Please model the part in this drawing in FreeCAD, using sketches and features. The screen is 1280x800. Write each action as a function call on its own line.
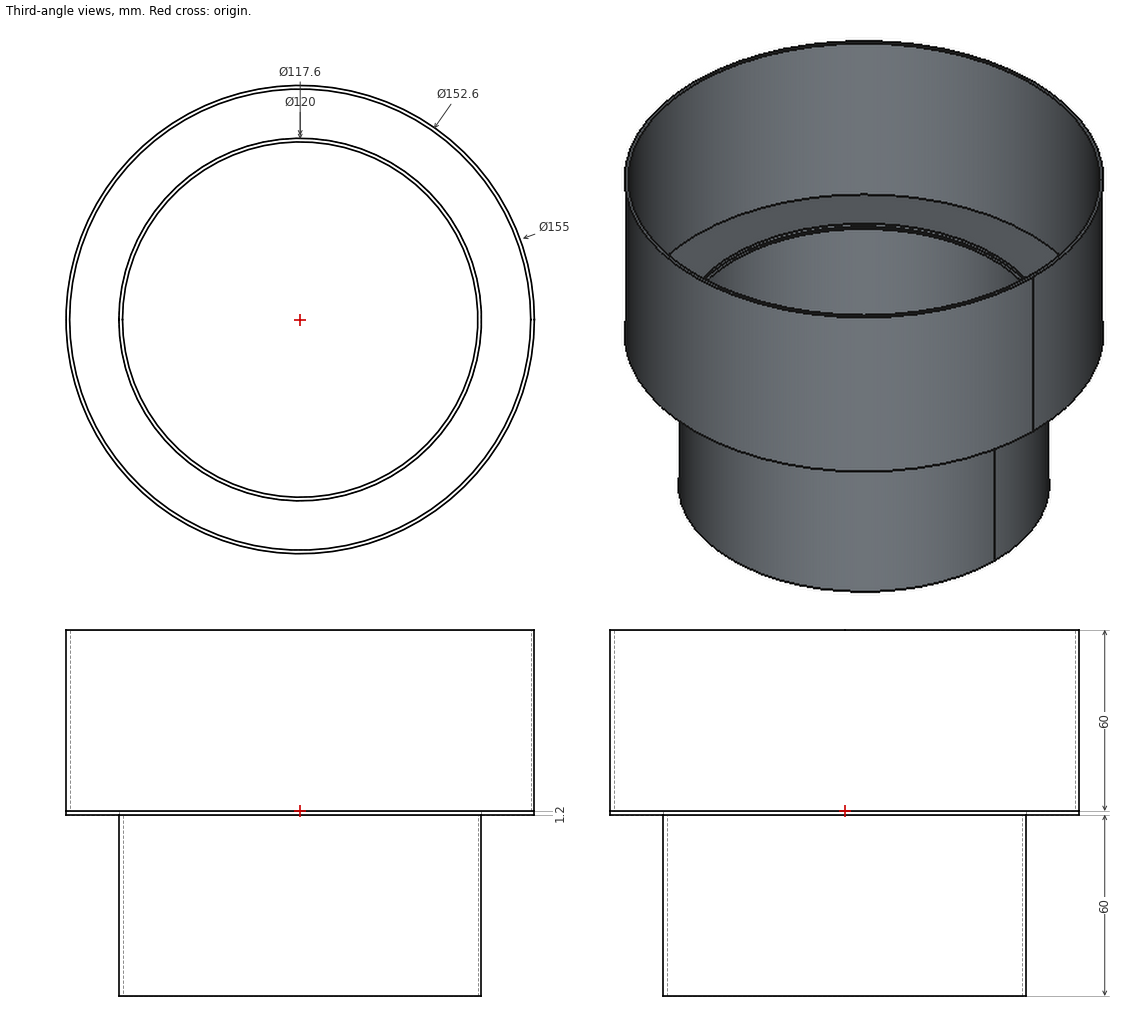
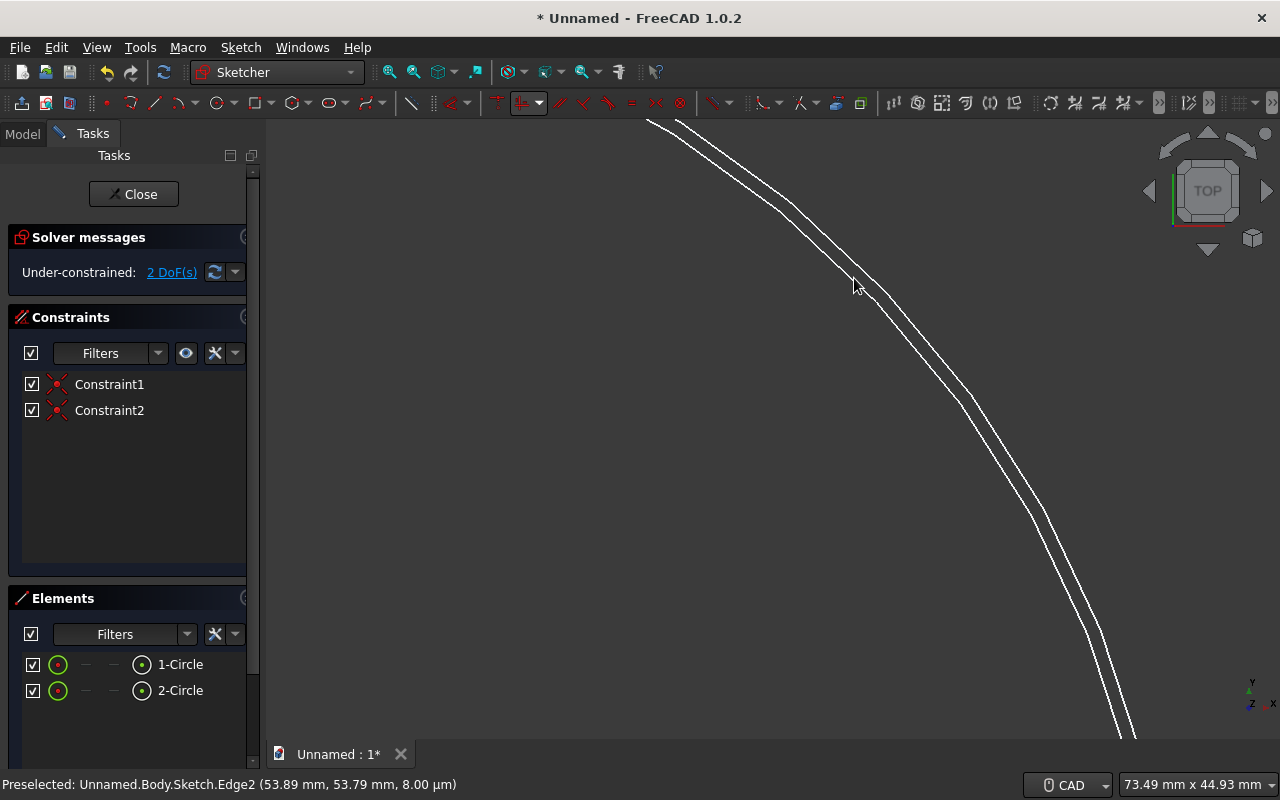
click(450, 104)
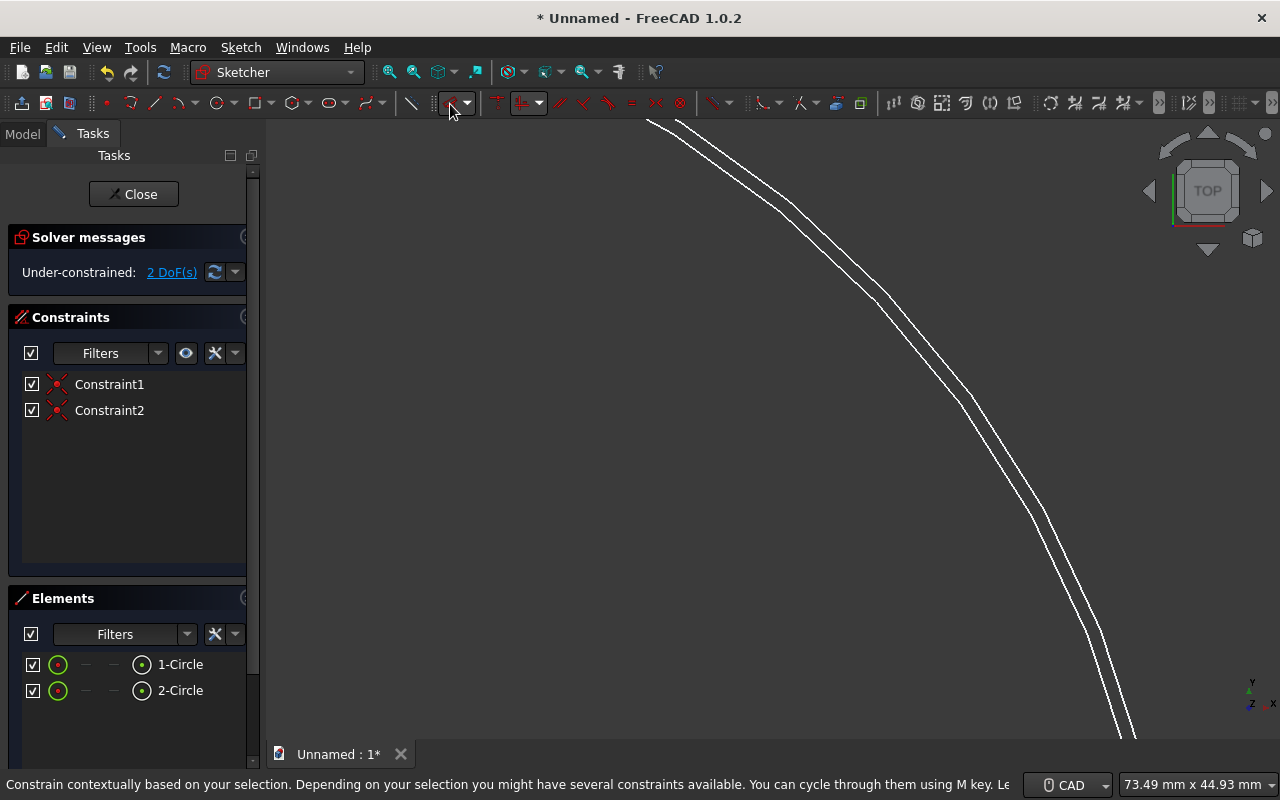
click(861, 266)
click(884, 243)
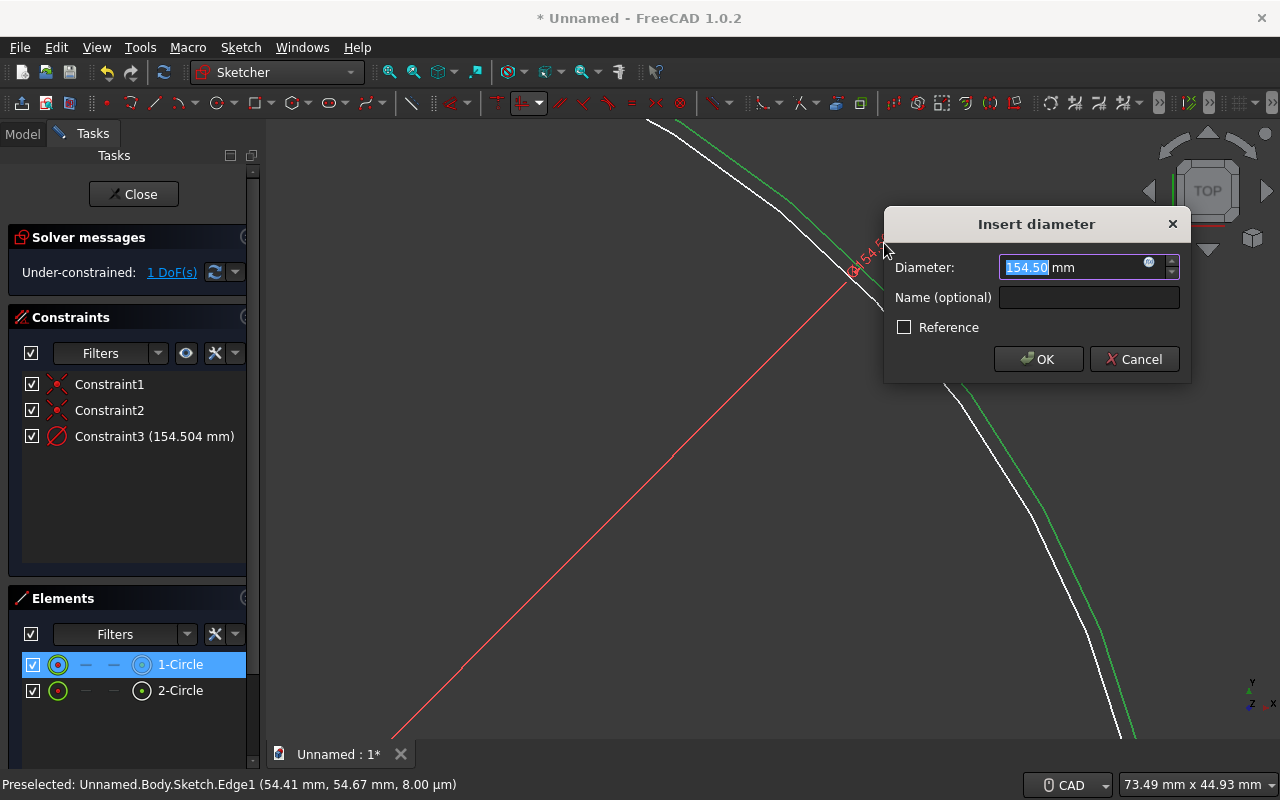
text(155)
key(Return)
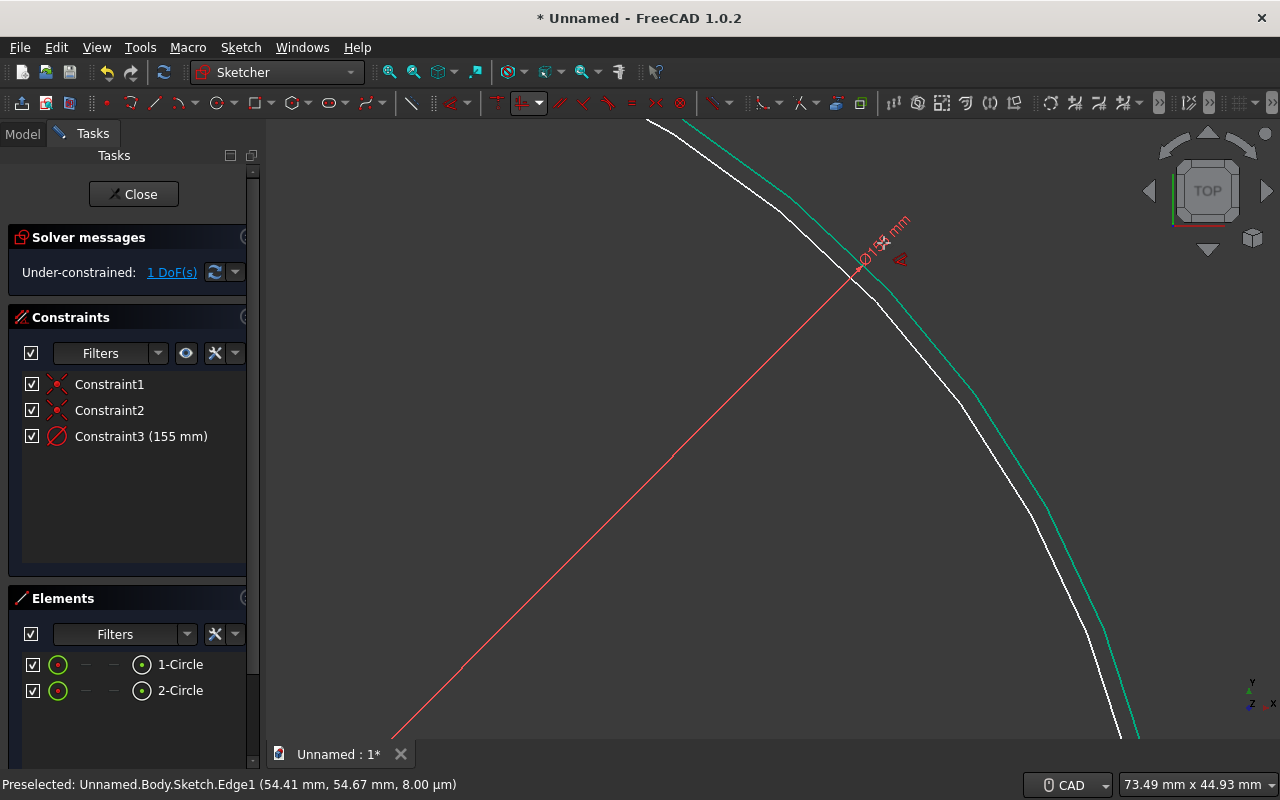
click(851, 276)
click(907, 219)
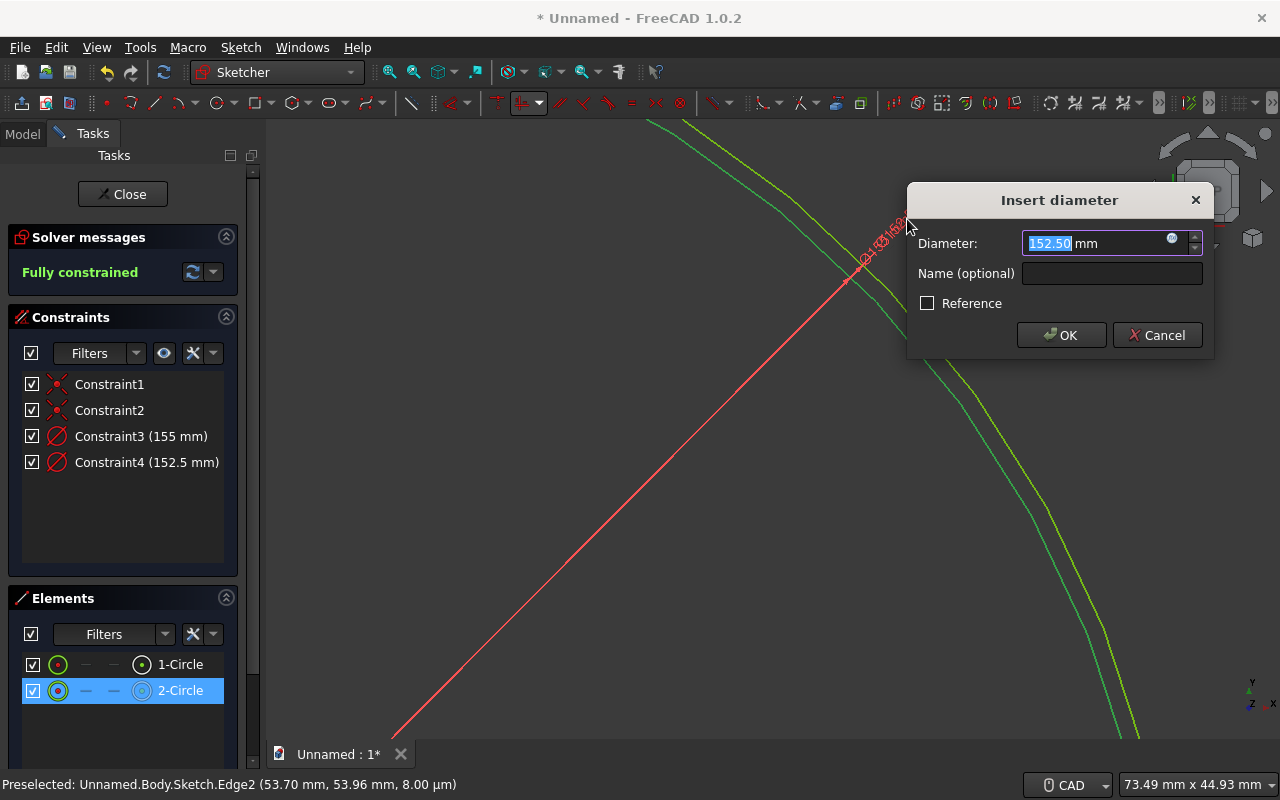
text(152.6)
key(Return)
key(Escape)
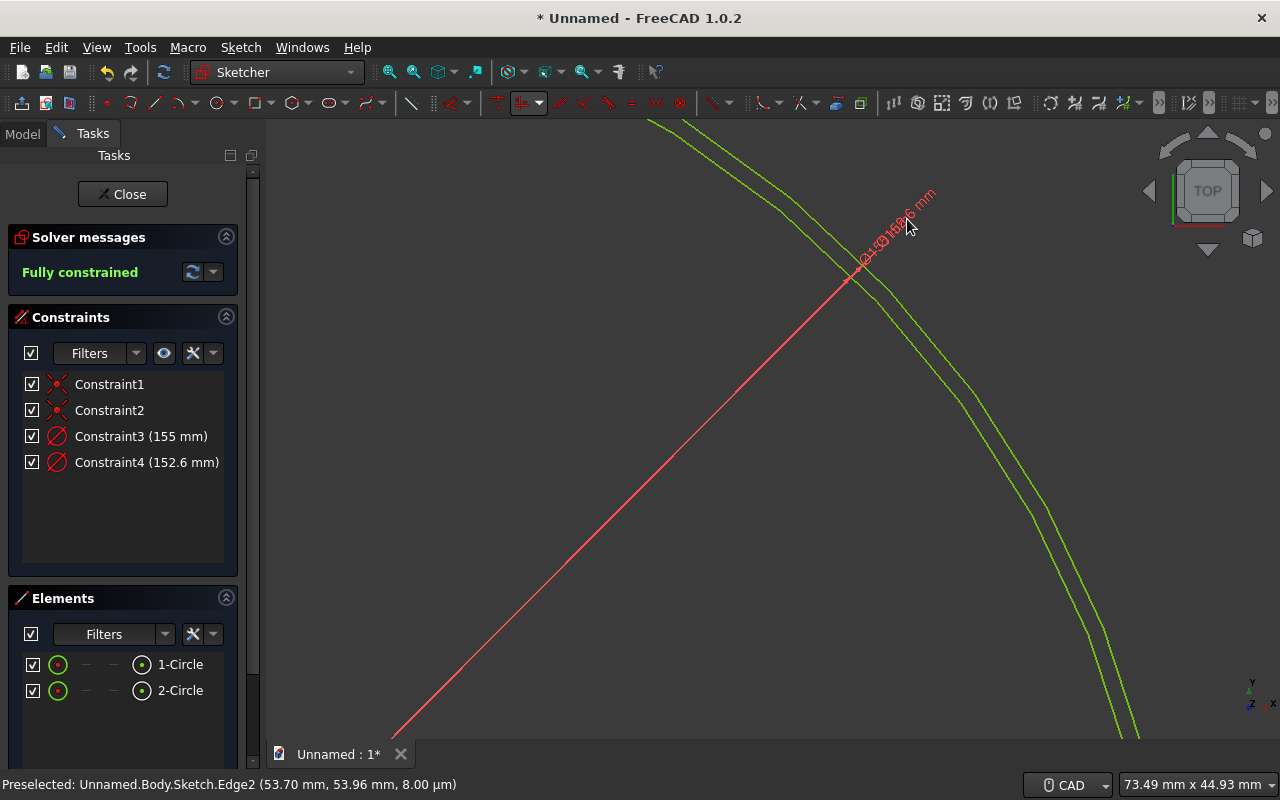
click(123, 194)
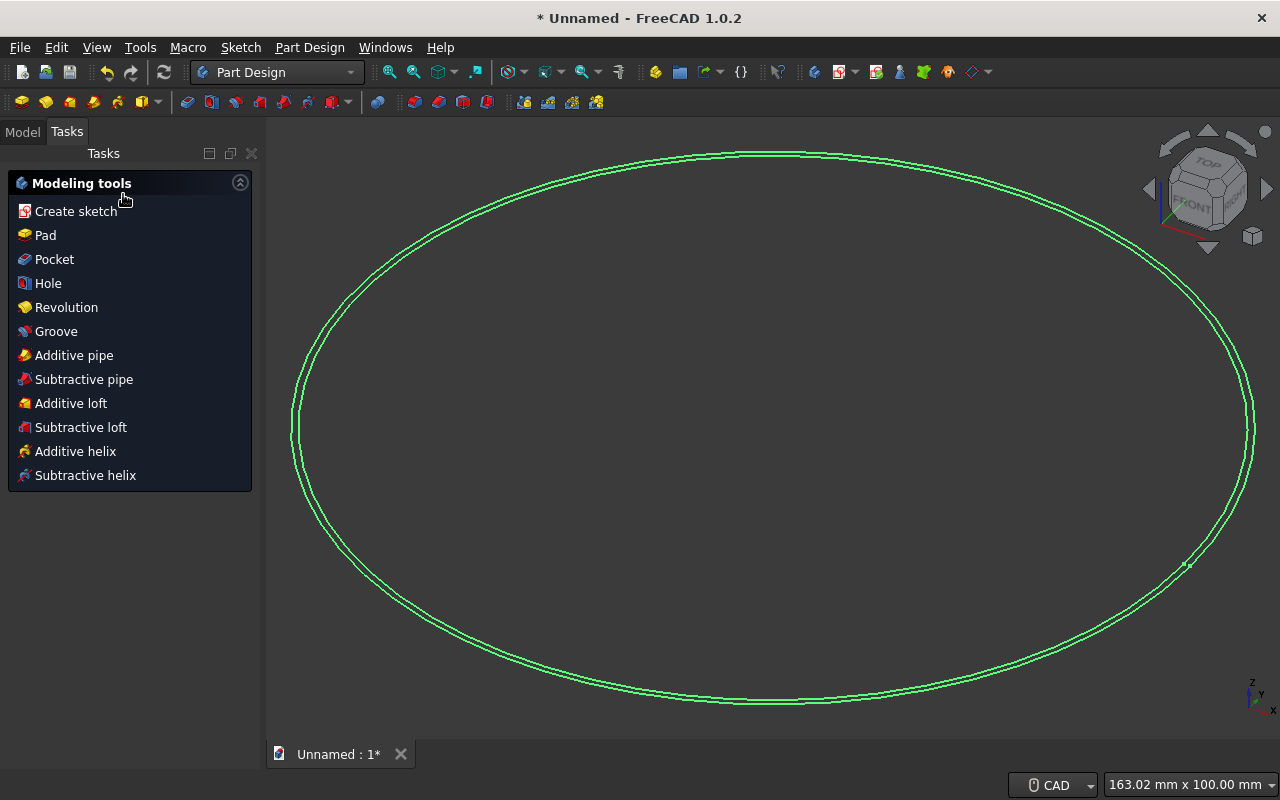
click(22, 102)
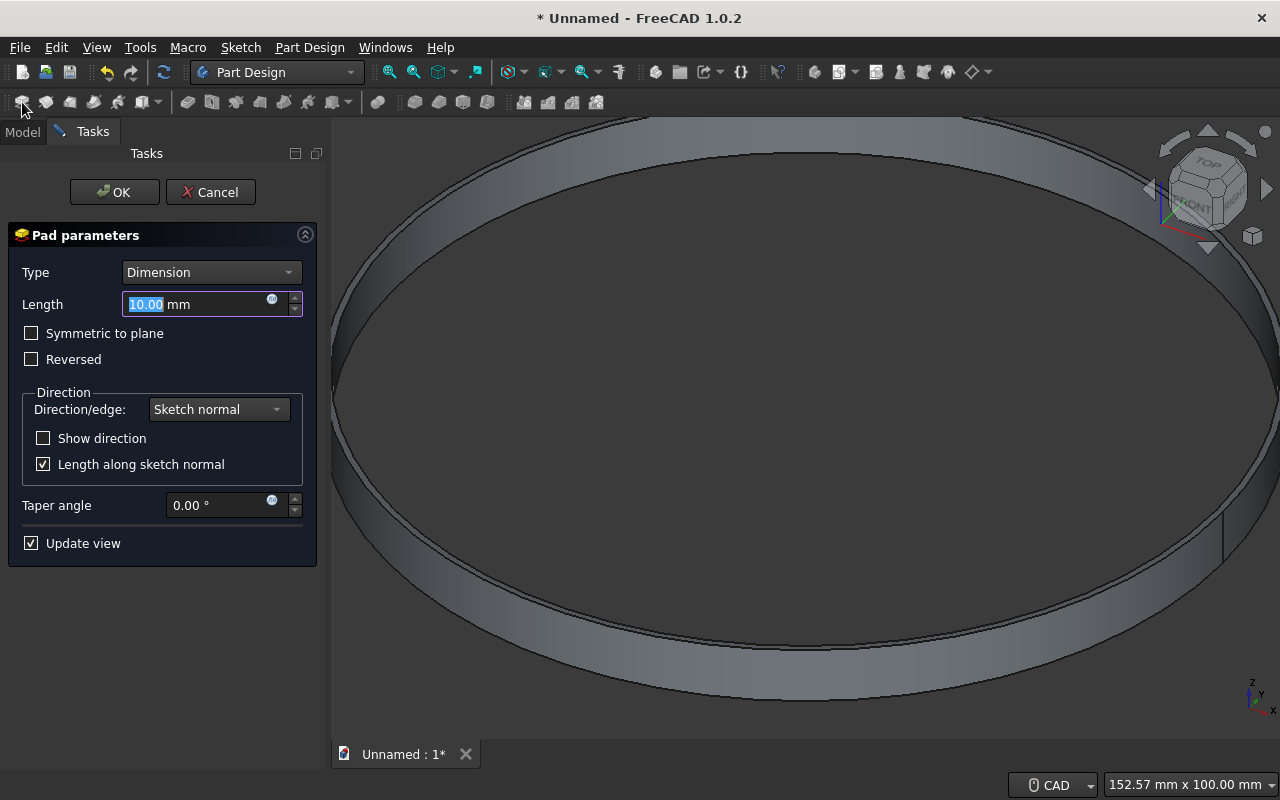
text(60)
key(Tab)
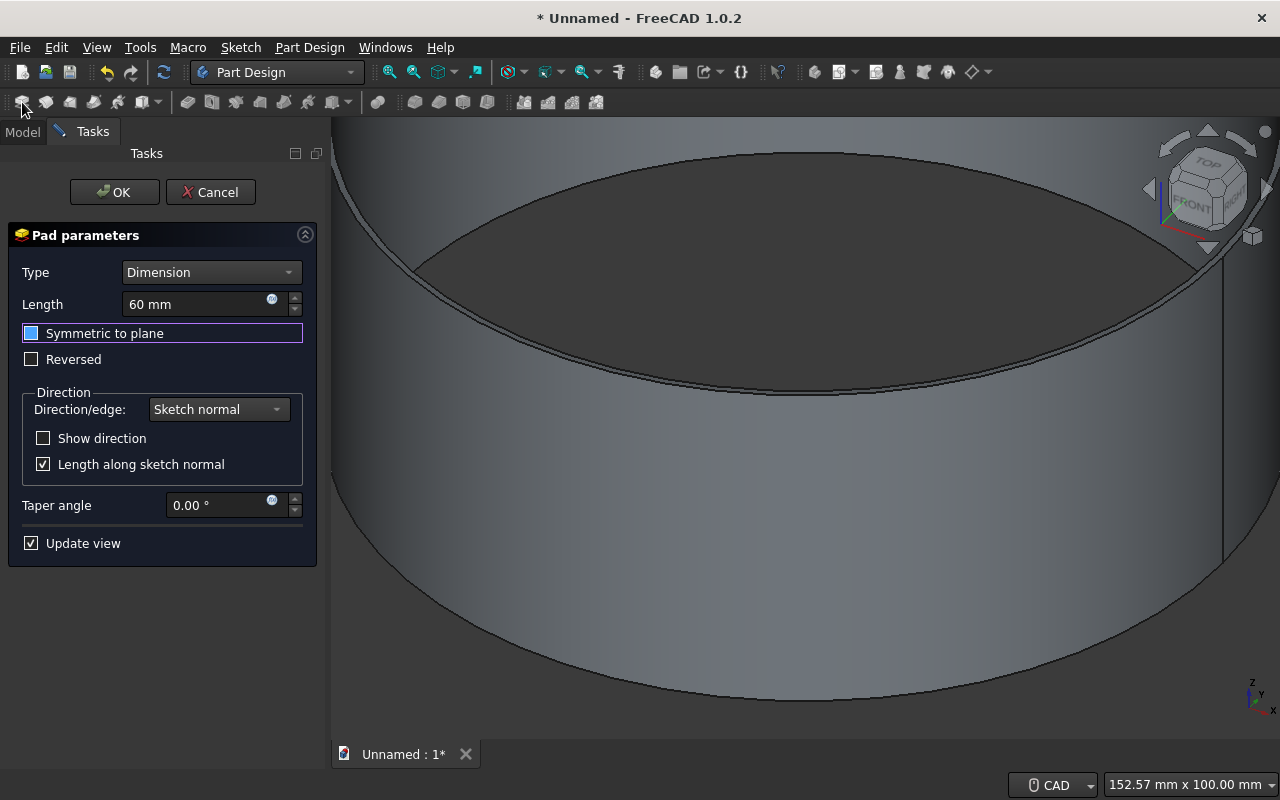
click(115, 192)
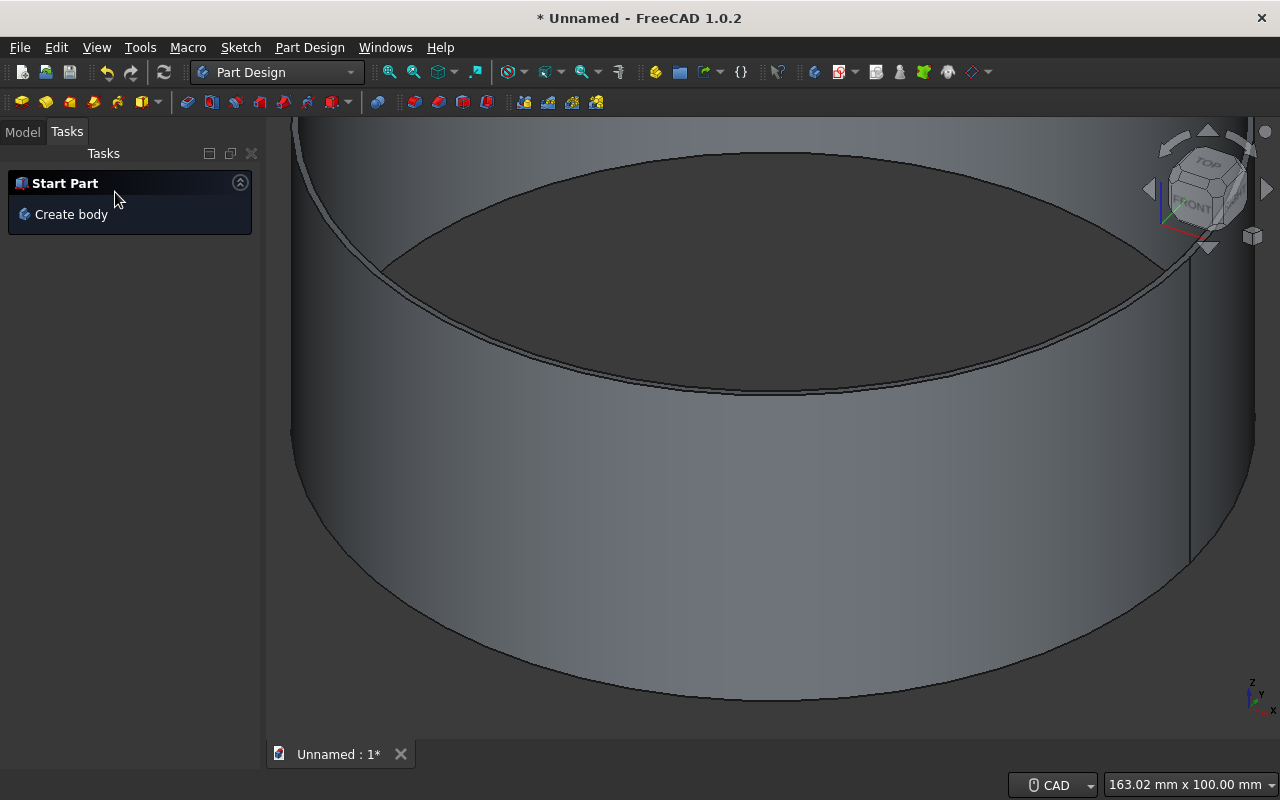
click(390, 72)